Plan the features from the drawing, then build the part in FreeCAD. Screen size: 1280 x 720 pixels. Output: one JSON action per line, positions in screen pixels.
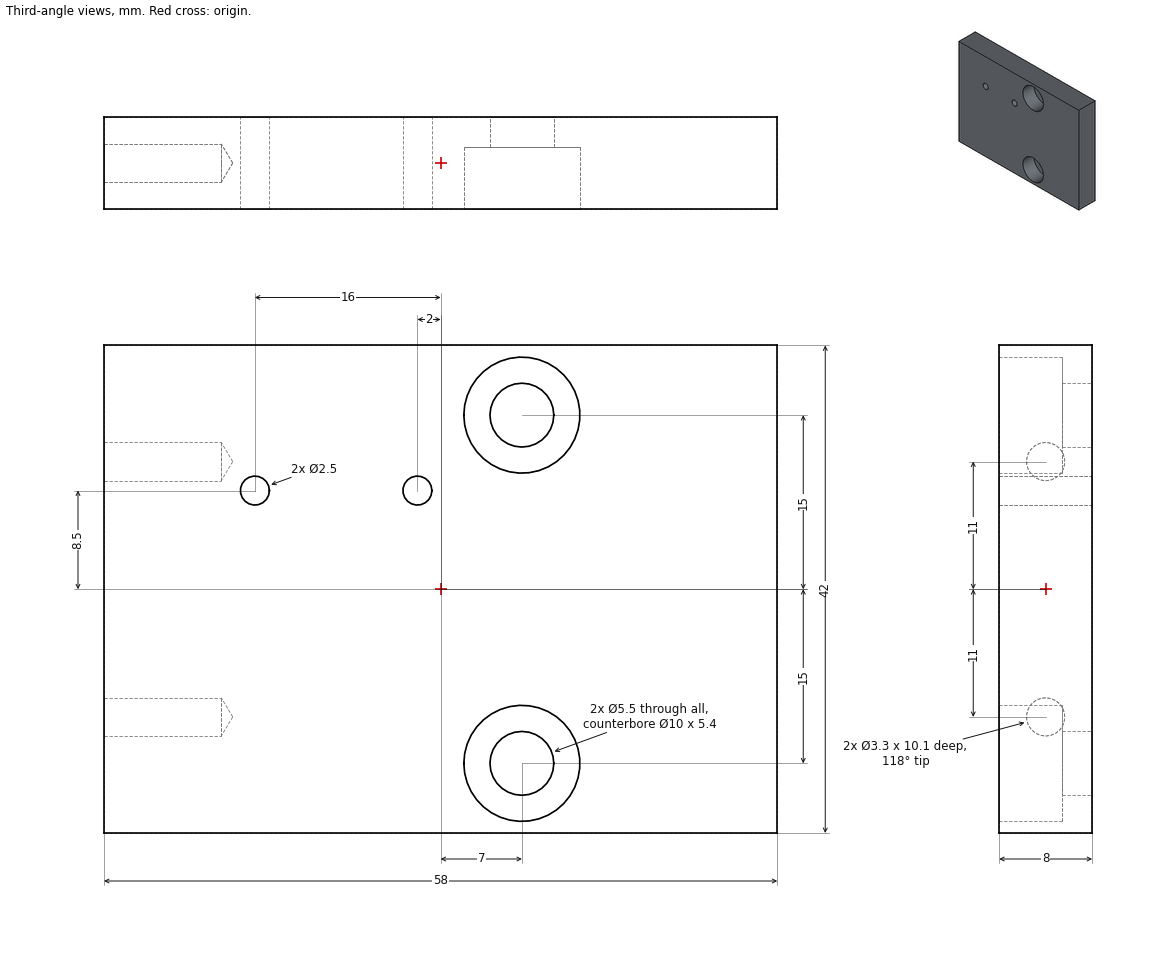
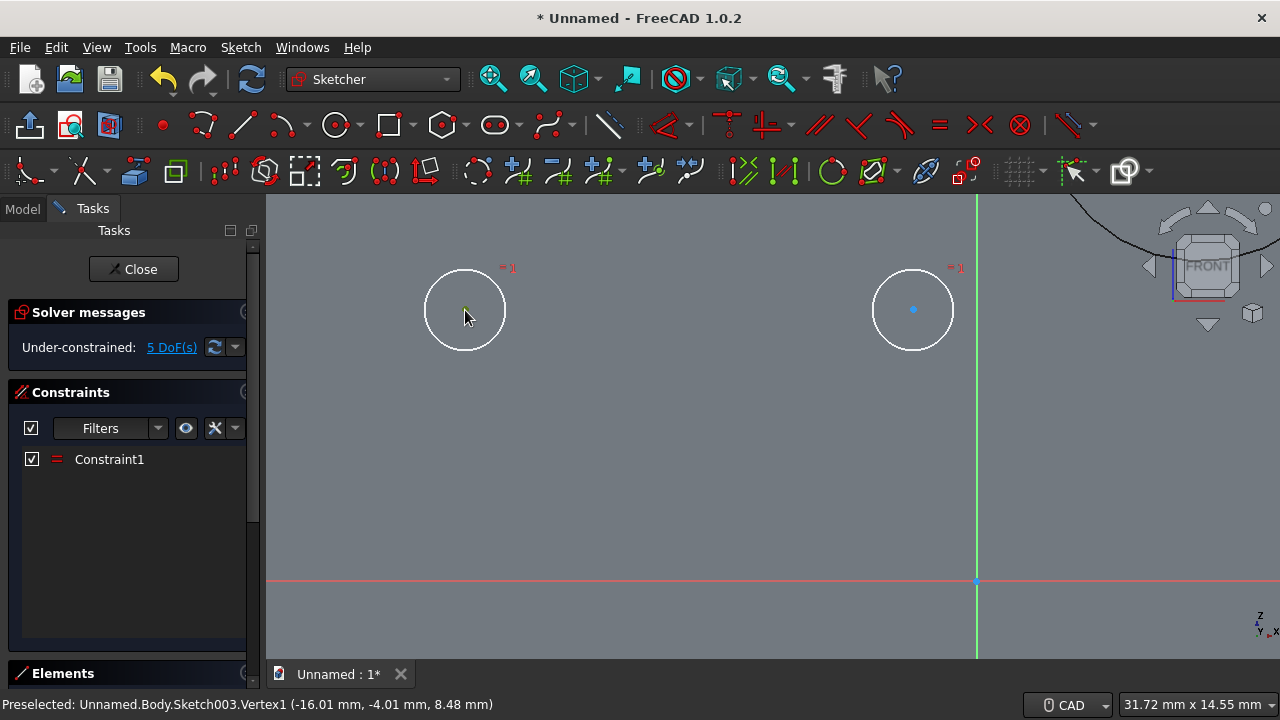
{"action": "left_click", "coordinate": [913, 310]}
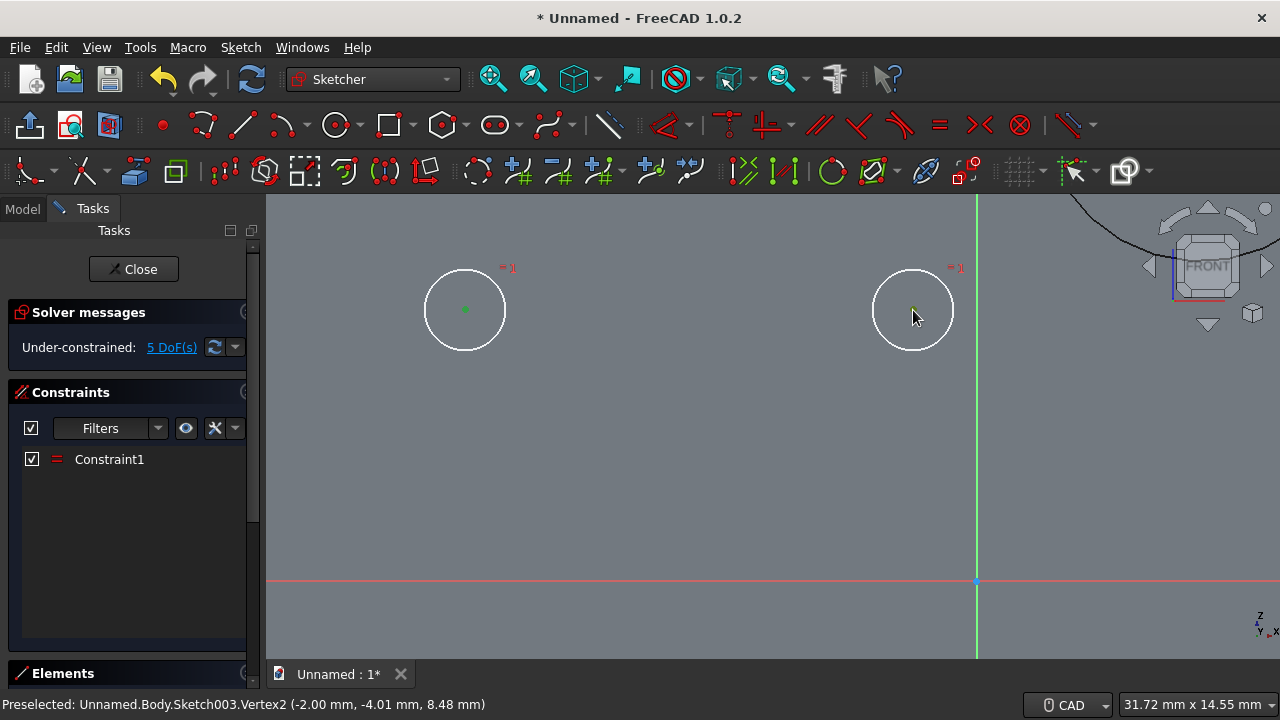
{"action": "left_click", "coordinate": [794, 126]}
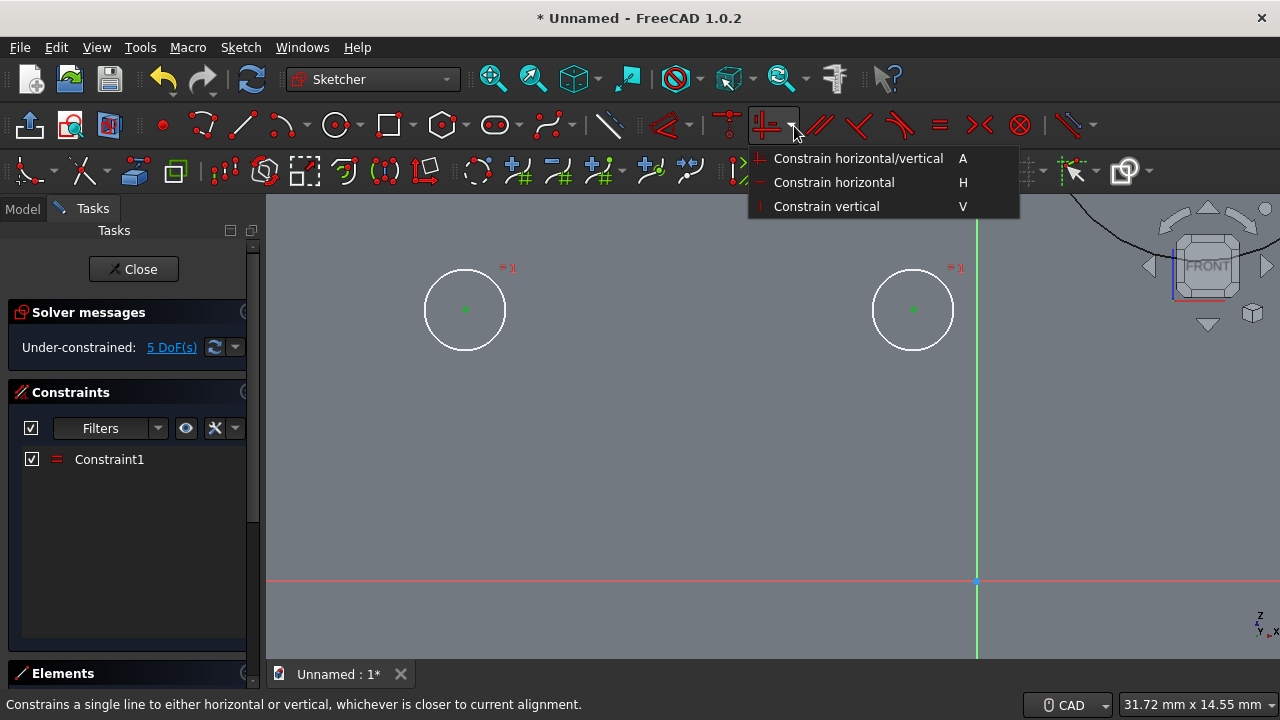
{"action": "left_click", "coordinate": [884, 182]}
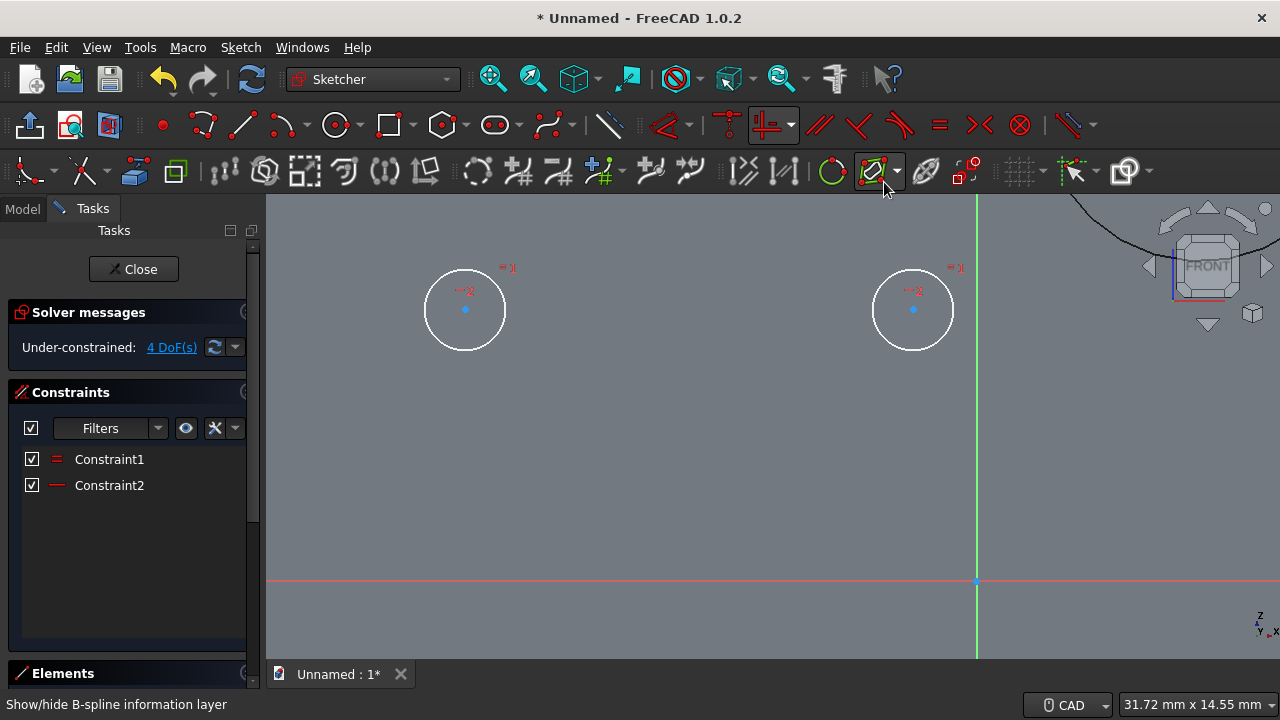
{"action": "left_click", "coordinate": [664, 126]}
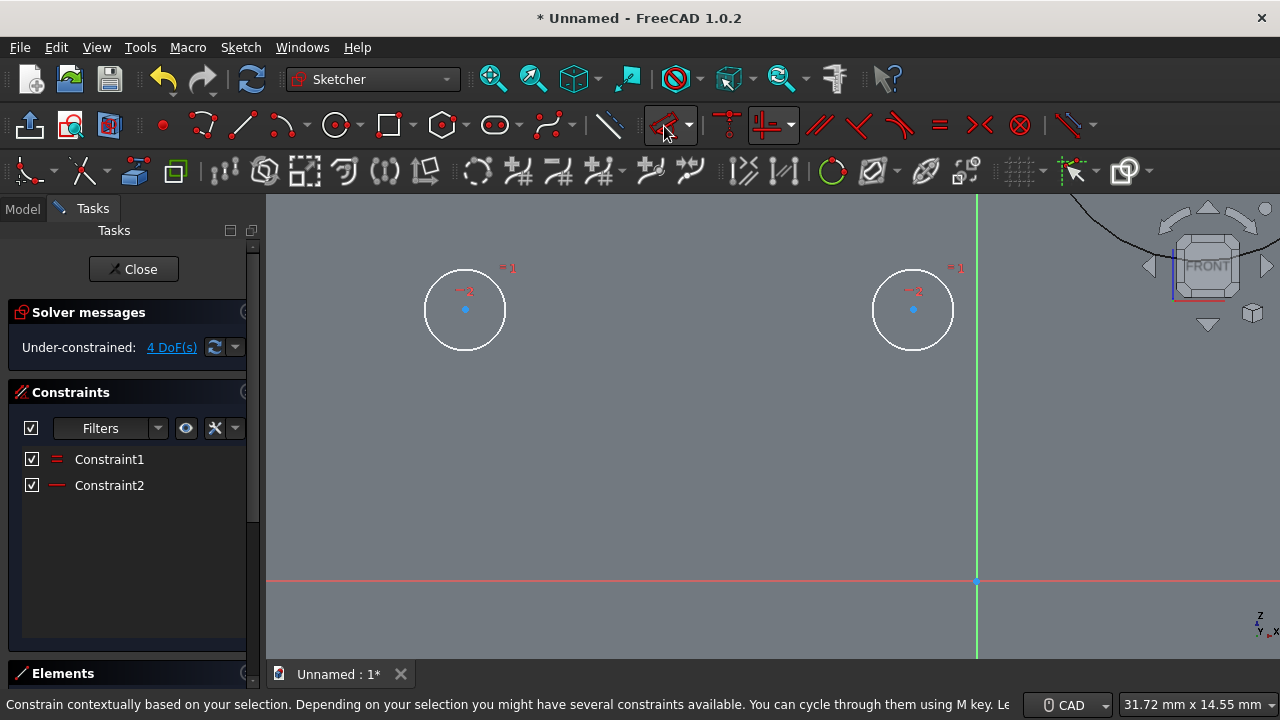
{"action": "left_click", "coordinate": [493, 281]}
{"action": "left_click", "coordinate": [515, 258]}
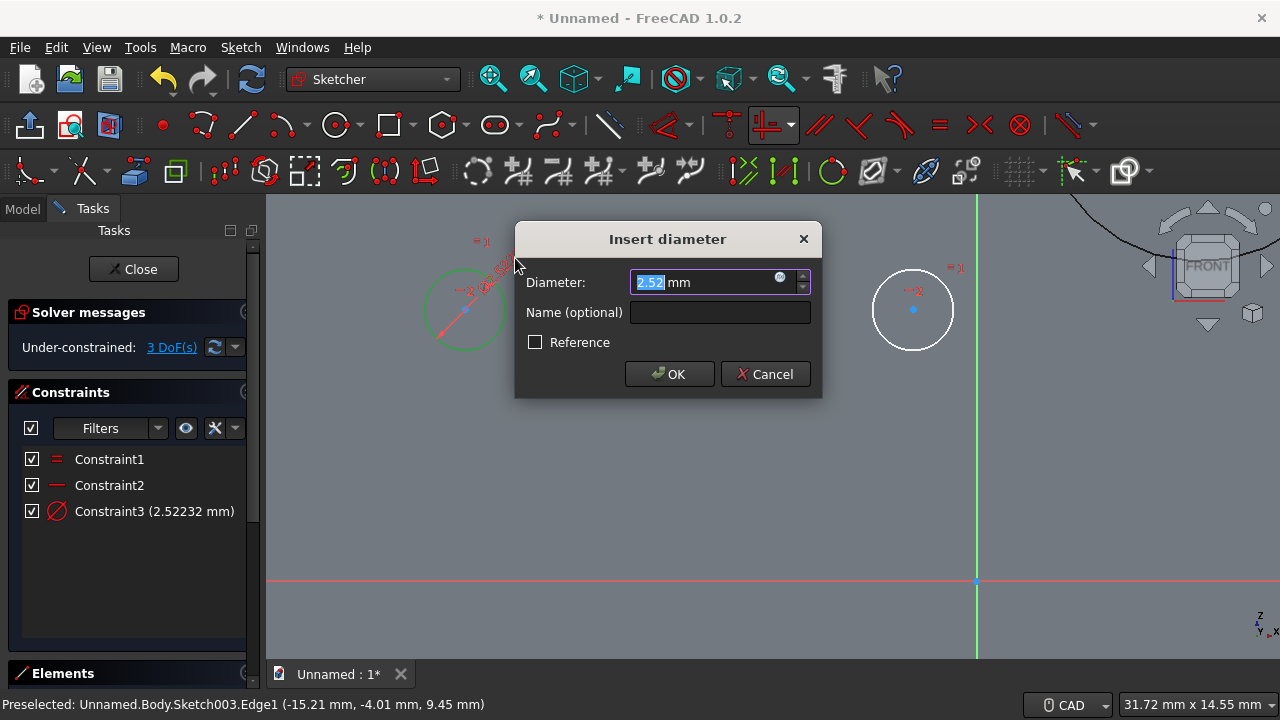
{"action": "type", "text": "2.5"}
{"action": "key", "text": "Return"}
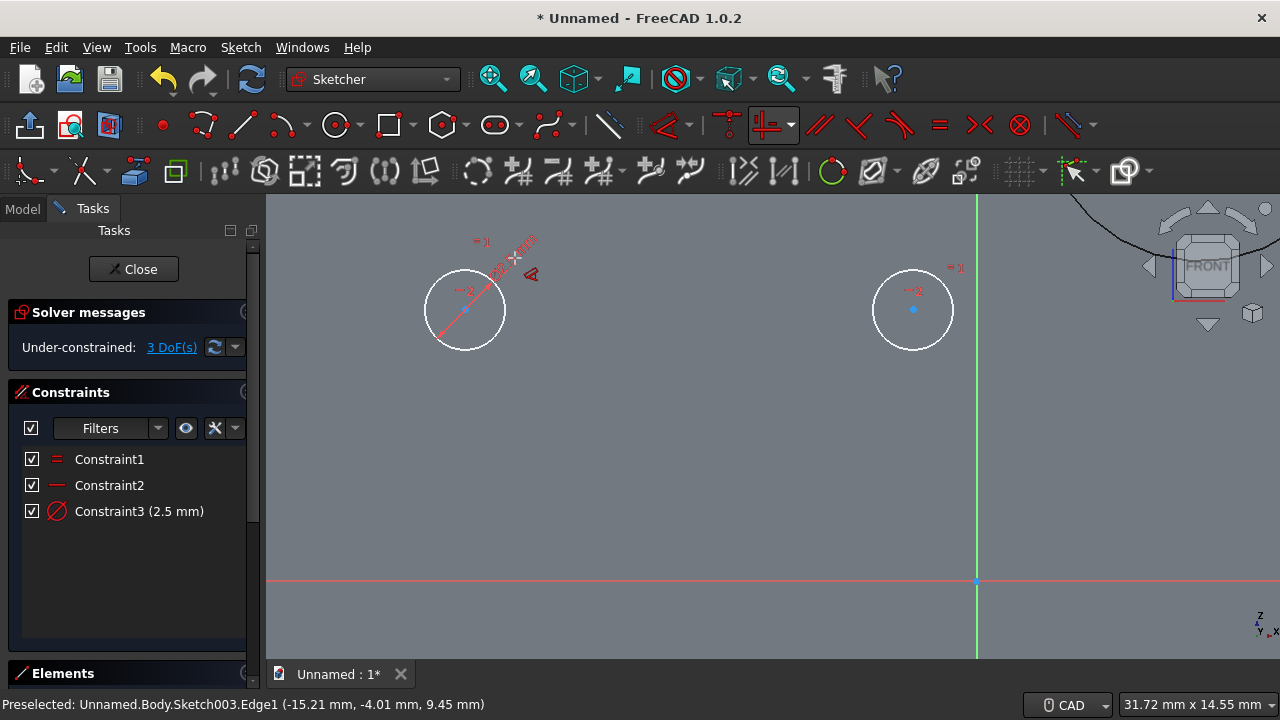
{"action": "left_click", "coordinate": [913, 310]}
{"action": "left_click", "coordinate": [945, 615]}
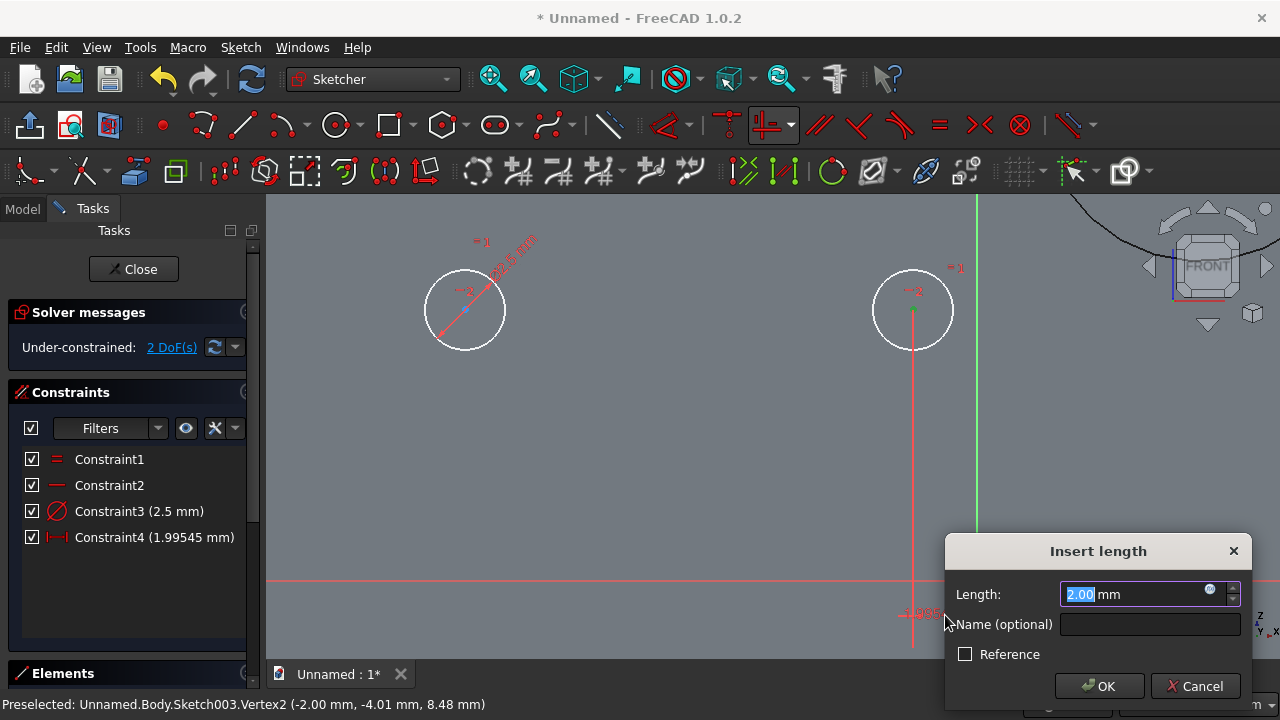
{"action": "type", "text": "2"}
{"action": "key", "text": "Return"}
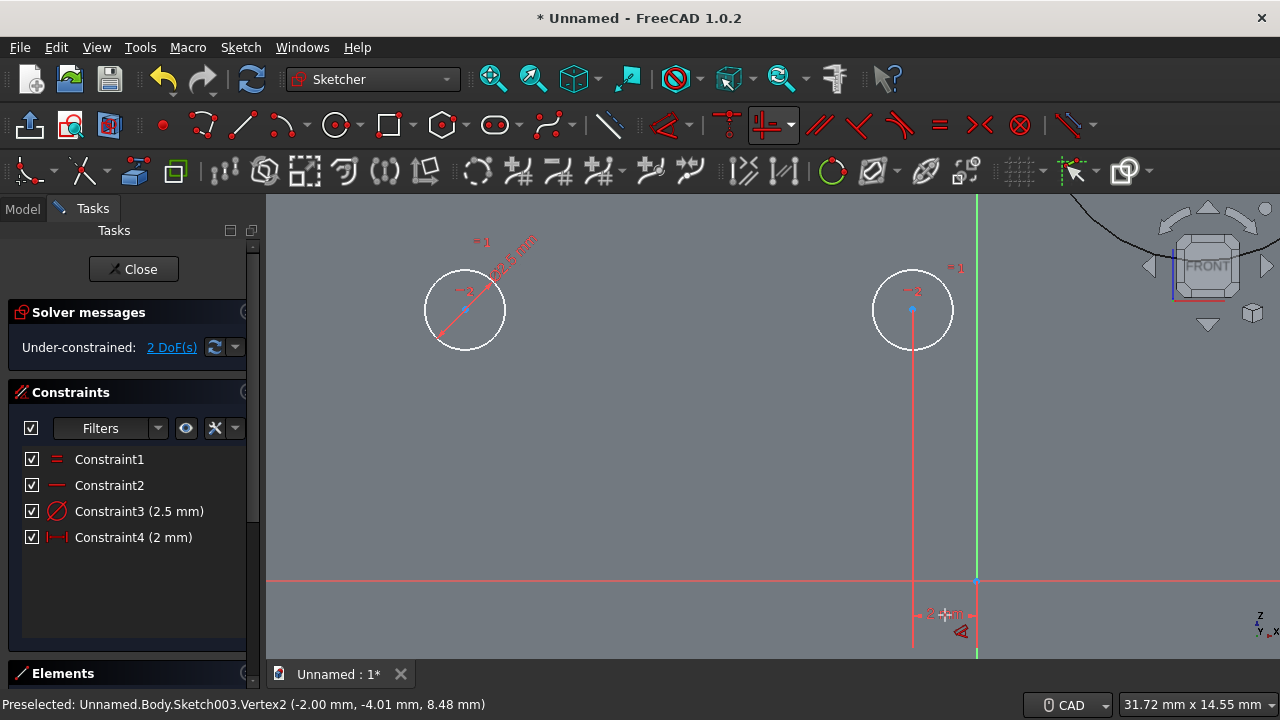
{"action": "left_click", "coordinate": [465, 310]}
{"action": "left_click", "coordinate": [721, 615]}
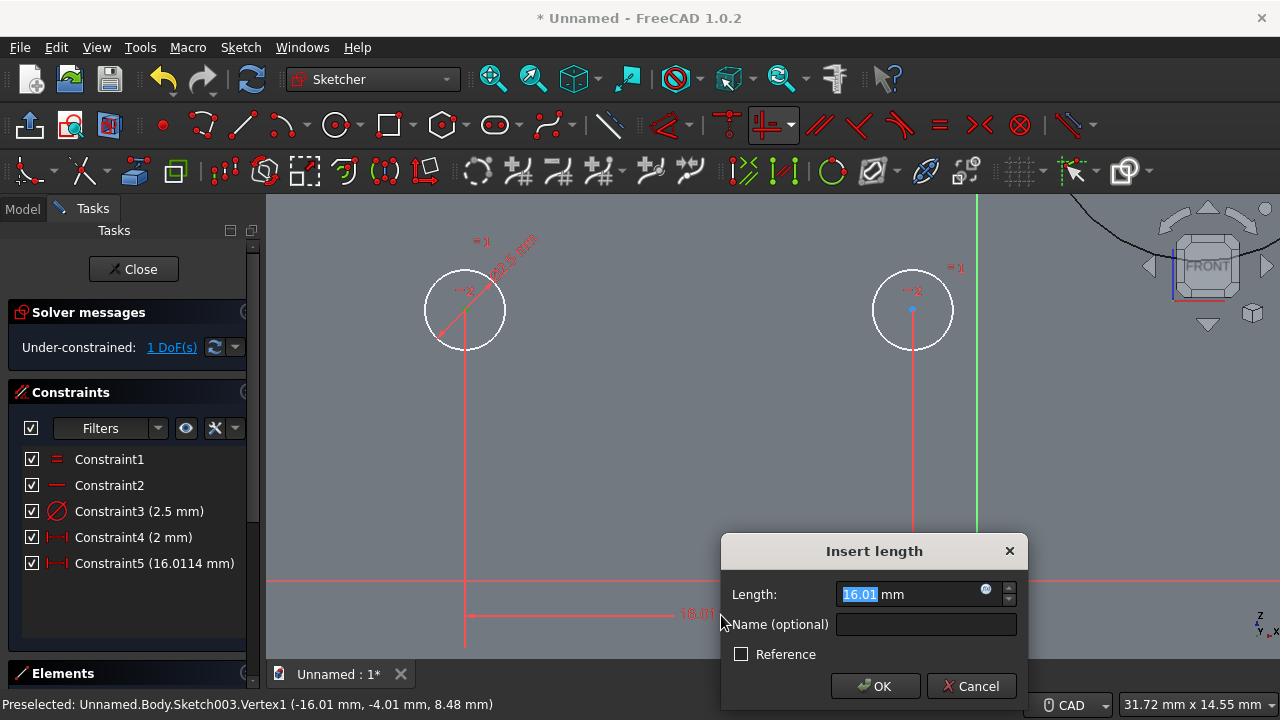
{"action": "type", "text": "16"}
{"action": "key", "text": "Return"}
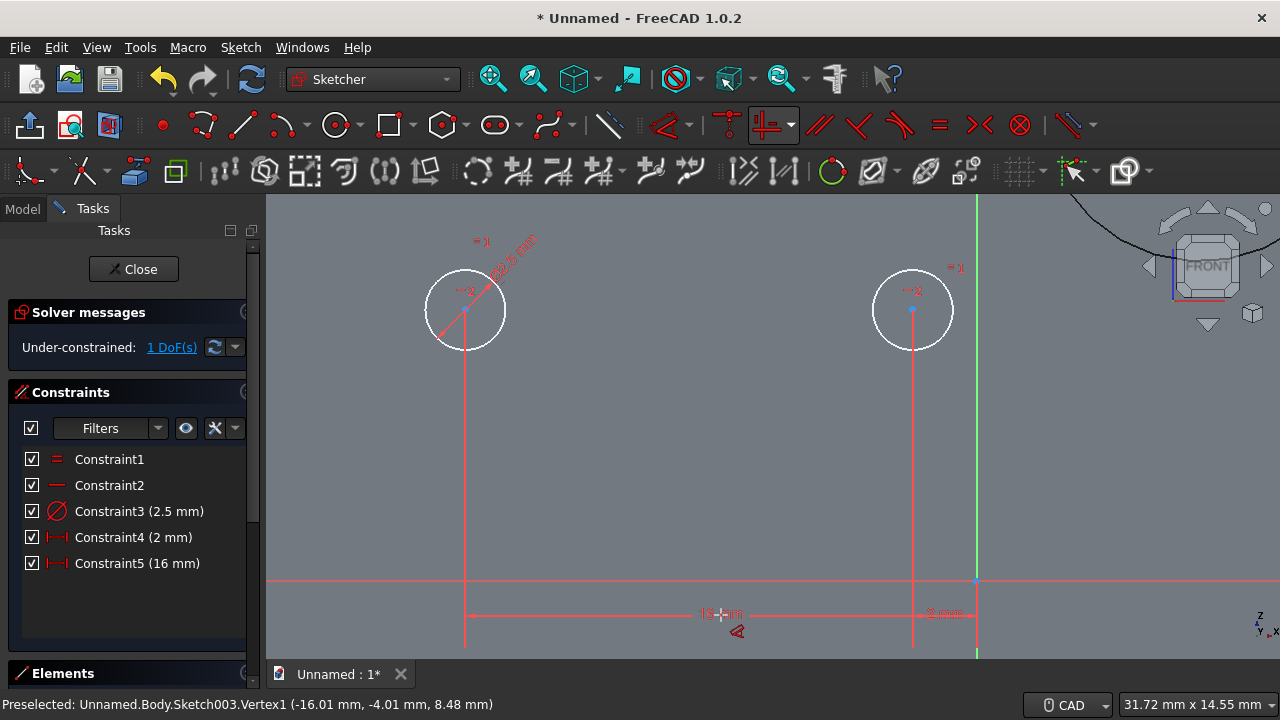
{"action": "left_click", "coordinate": [465, 310]}
{"action": "left_click", "coordinate": [1011, 446]}